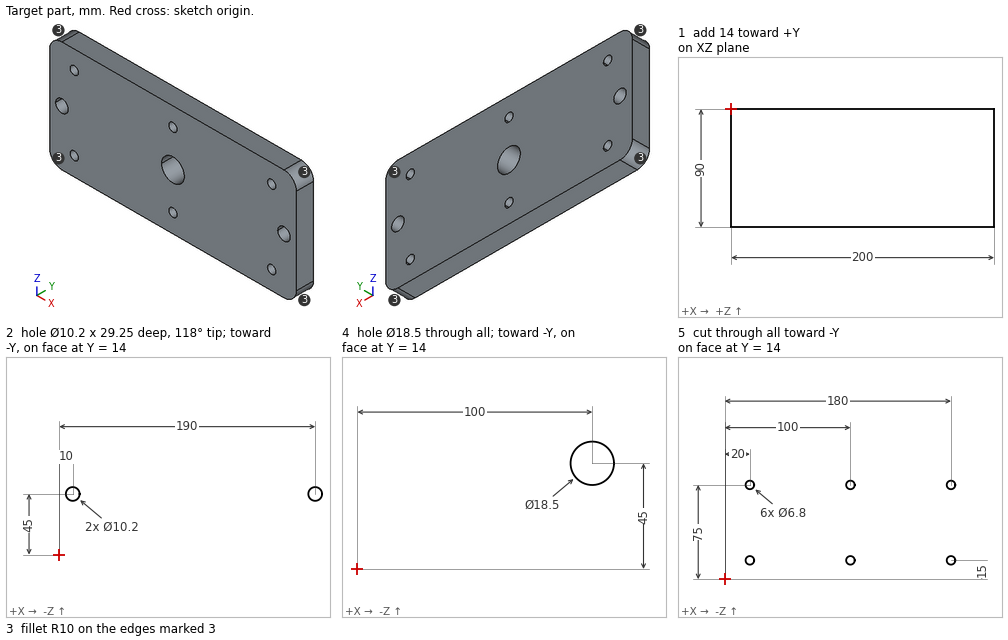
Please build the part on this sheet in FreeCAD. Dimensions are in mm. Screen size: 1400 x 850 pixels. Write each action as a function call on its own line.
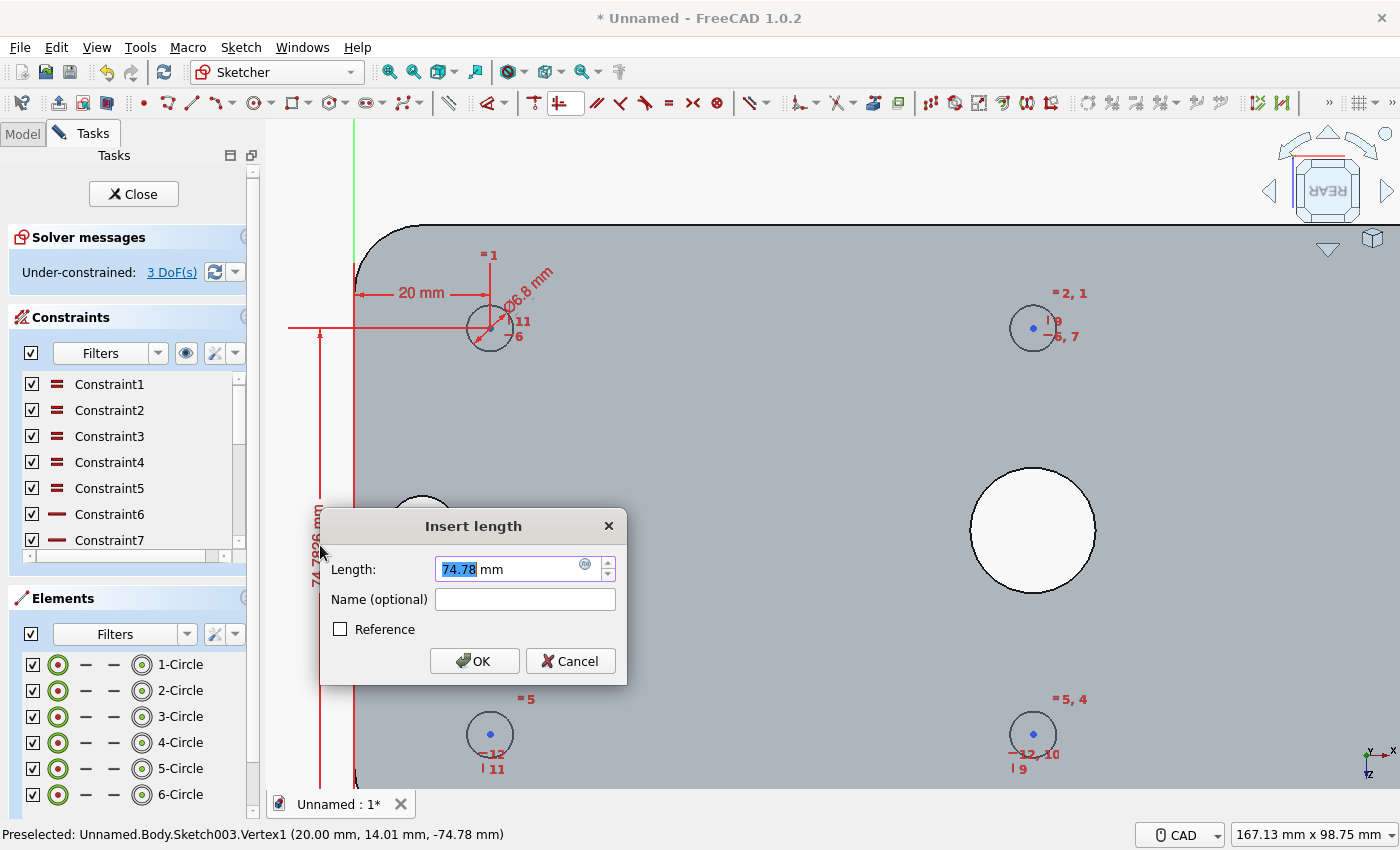
text(75)
key(Return)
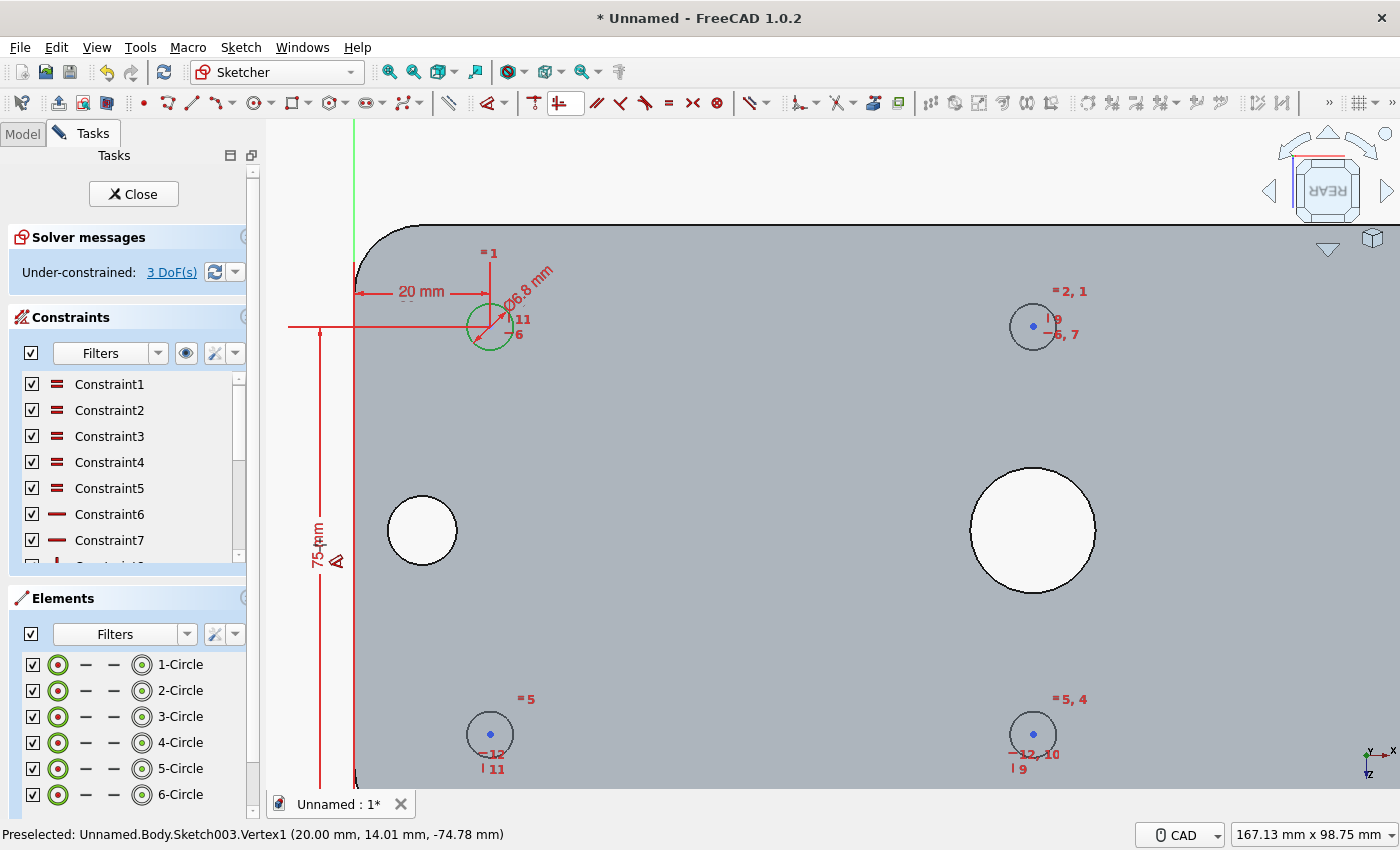
scroll(506, 313, down, 3)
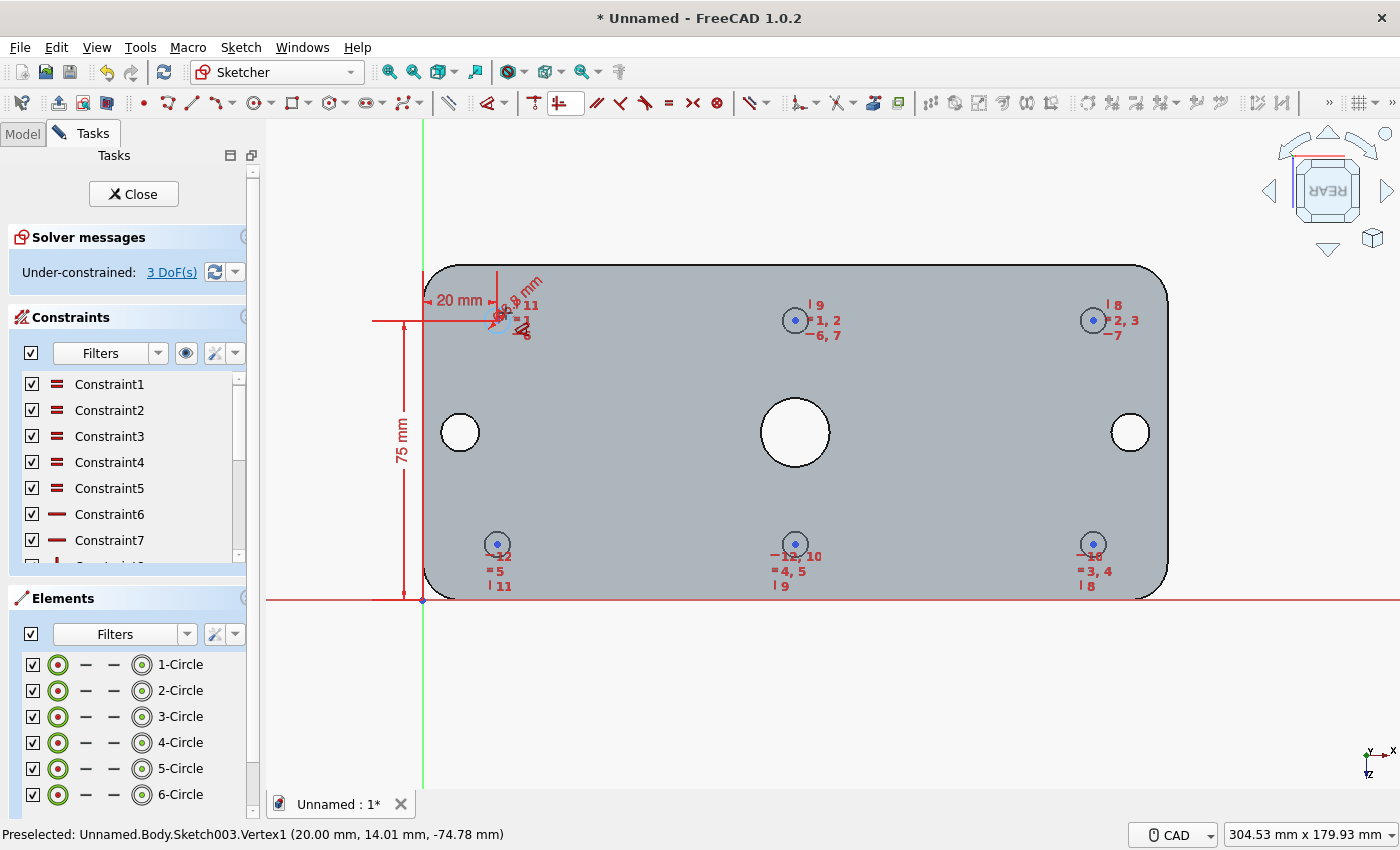
click(1093, 545)
click(389, 572)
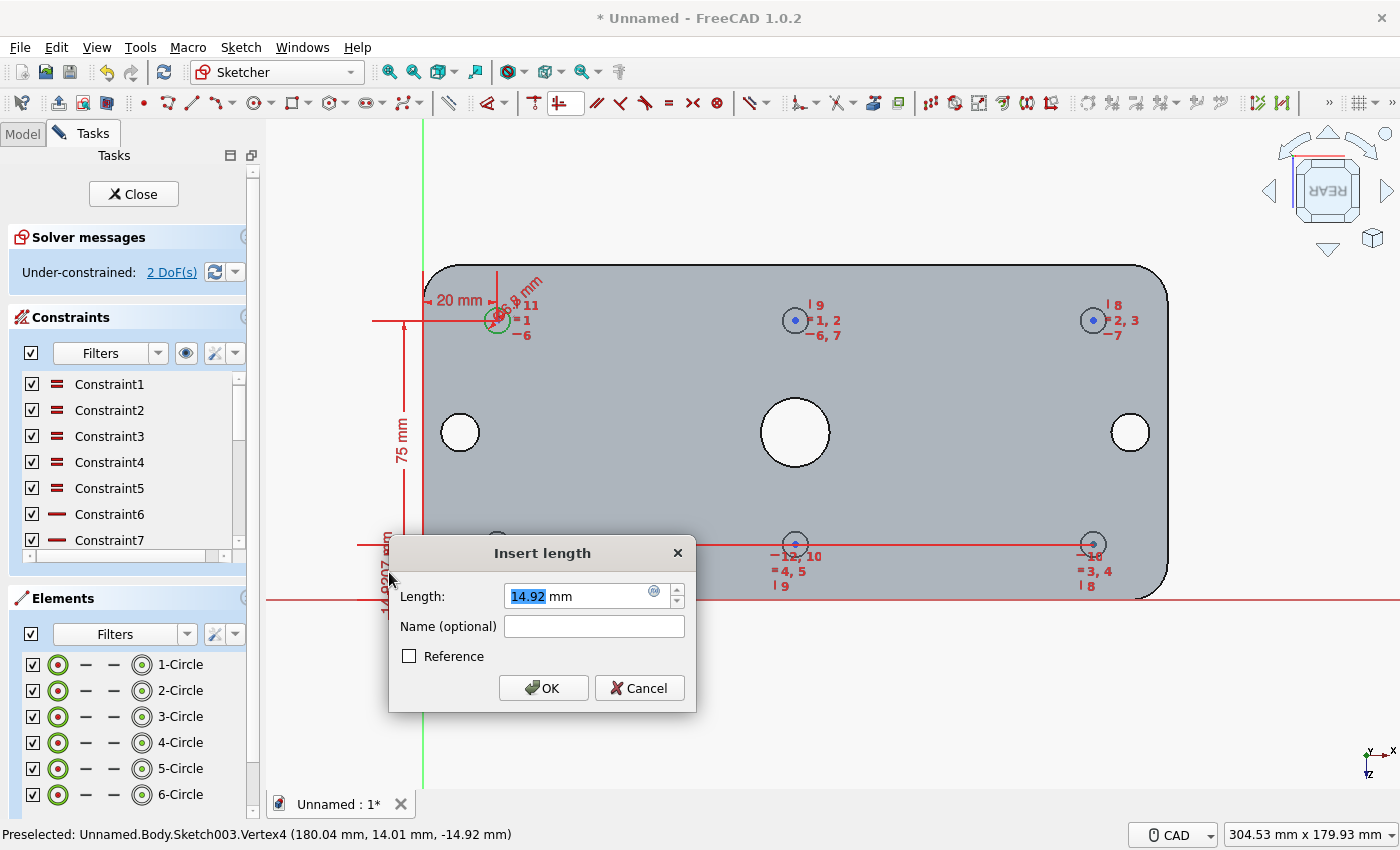
text(15)
key(Return)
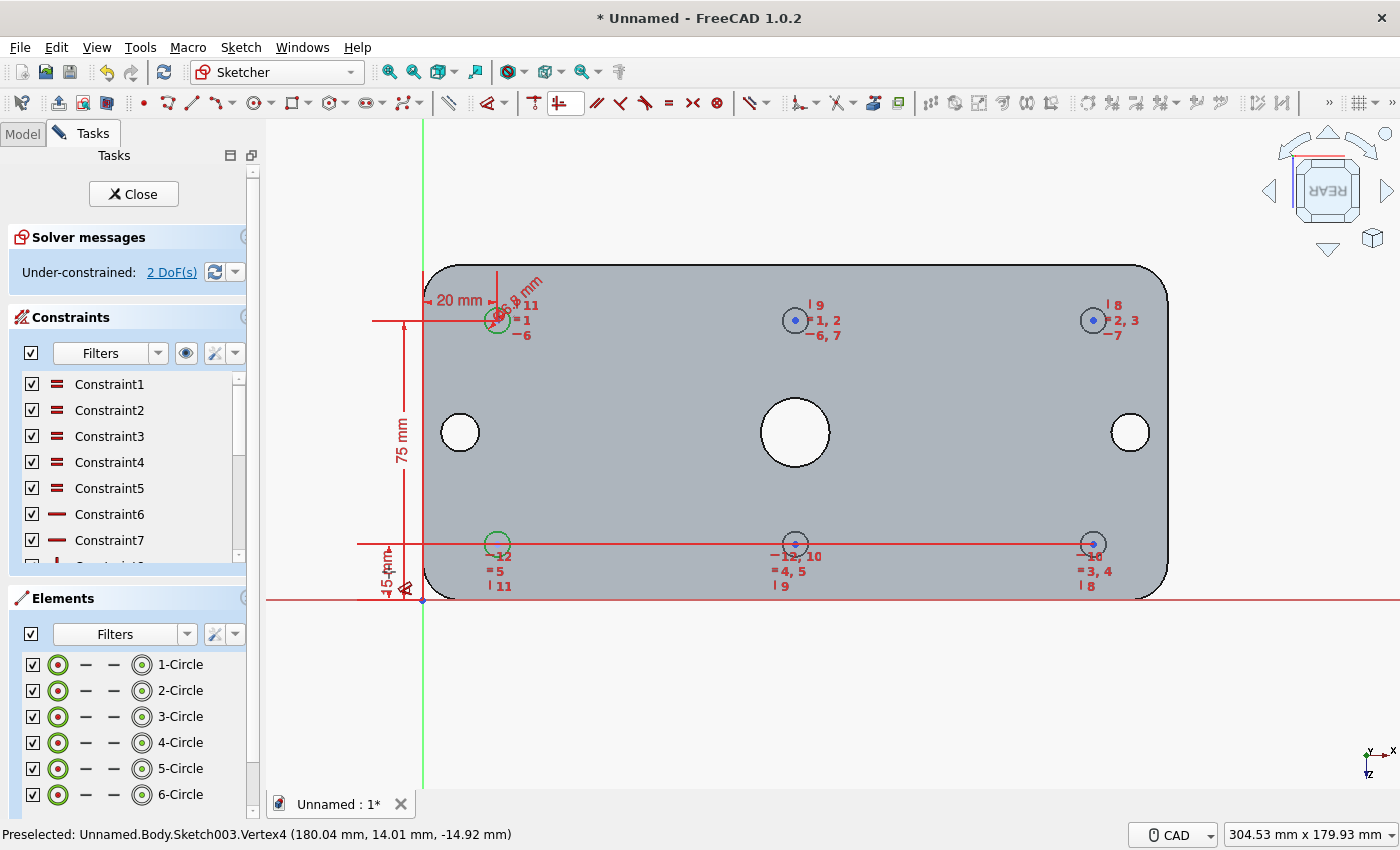
click(795, 321)
click(609, 634)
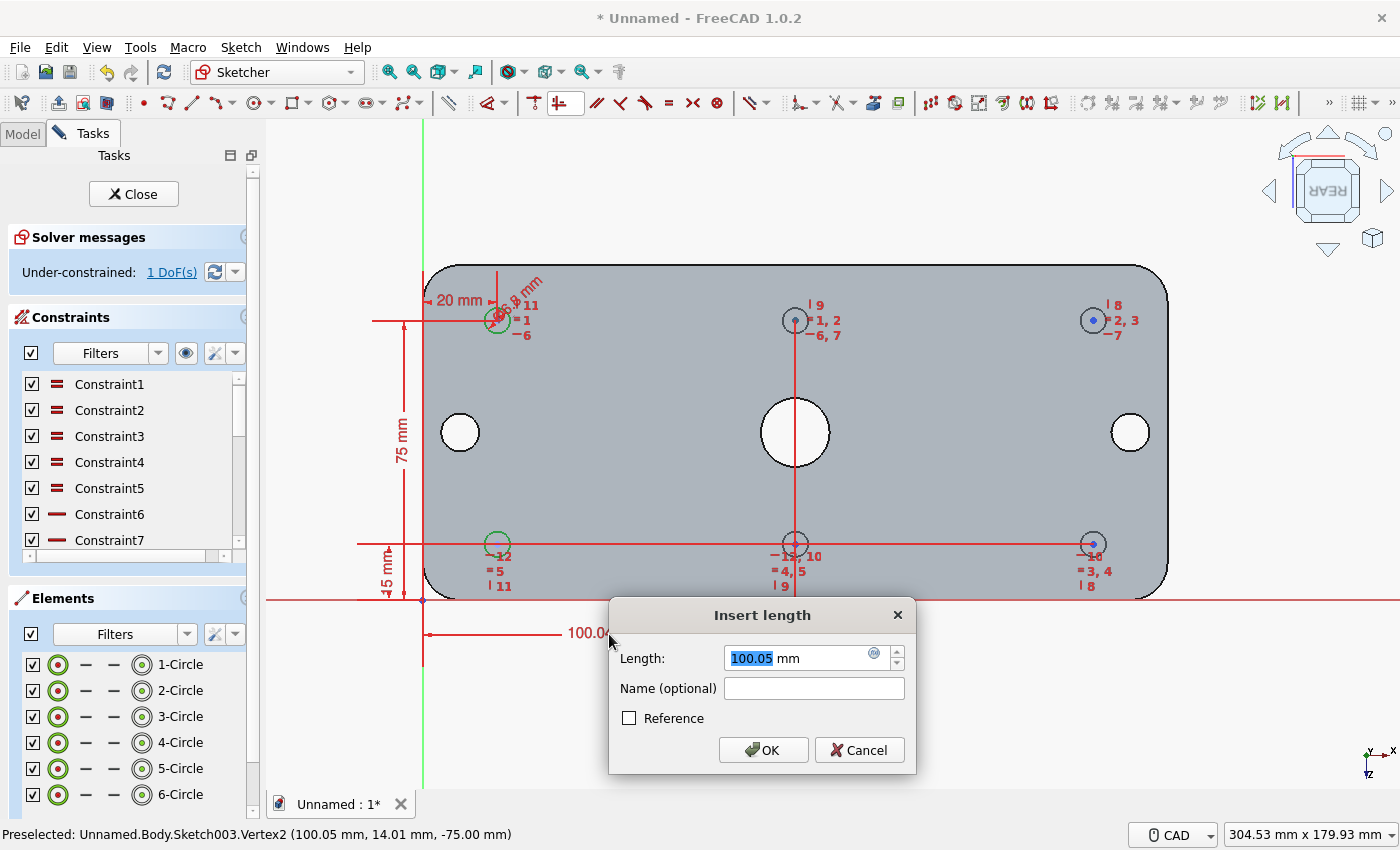
text(100)
key(Return)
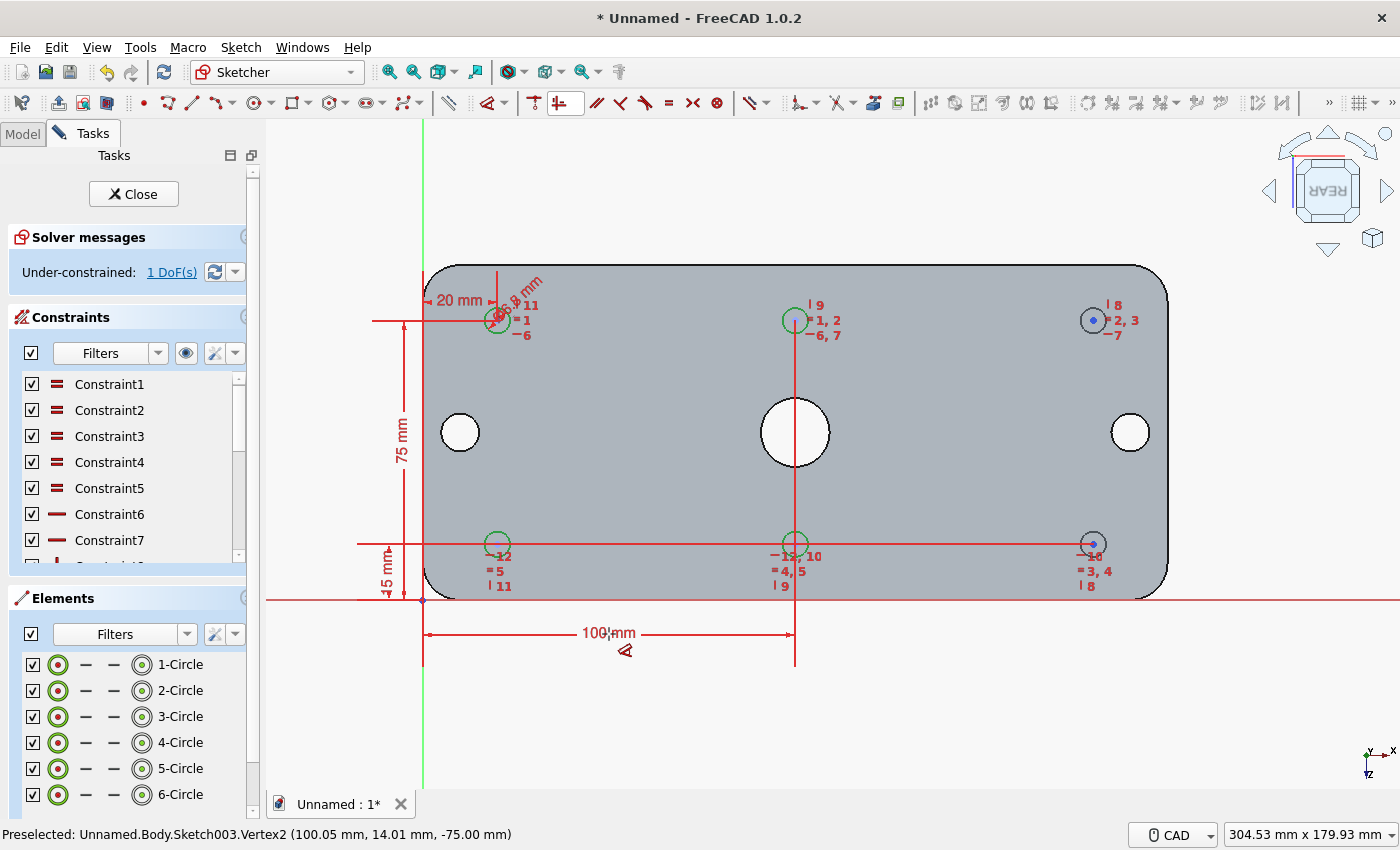
click(1093, 321)
click(758, 634)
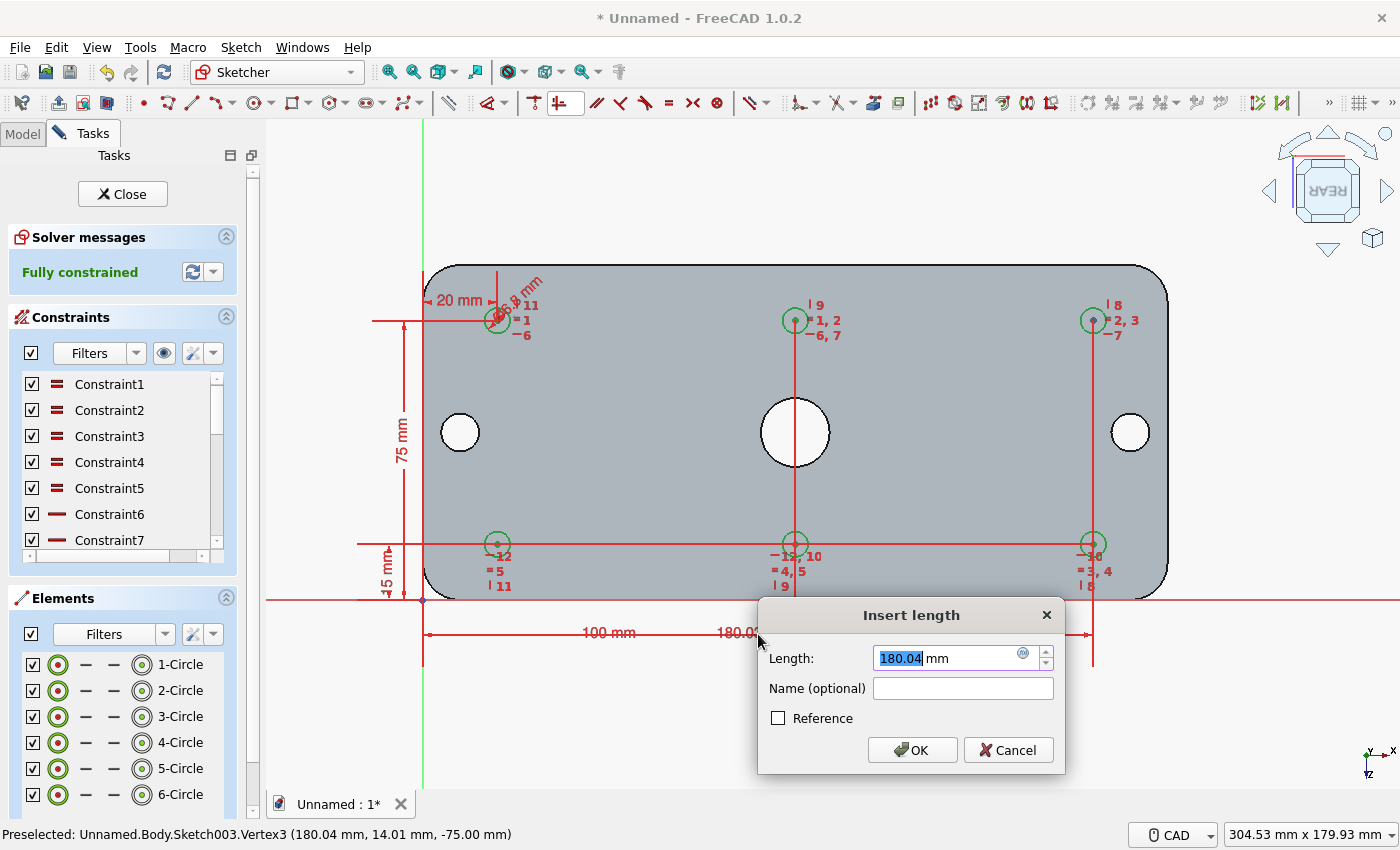
text(180)
key(Return)
key(Escape)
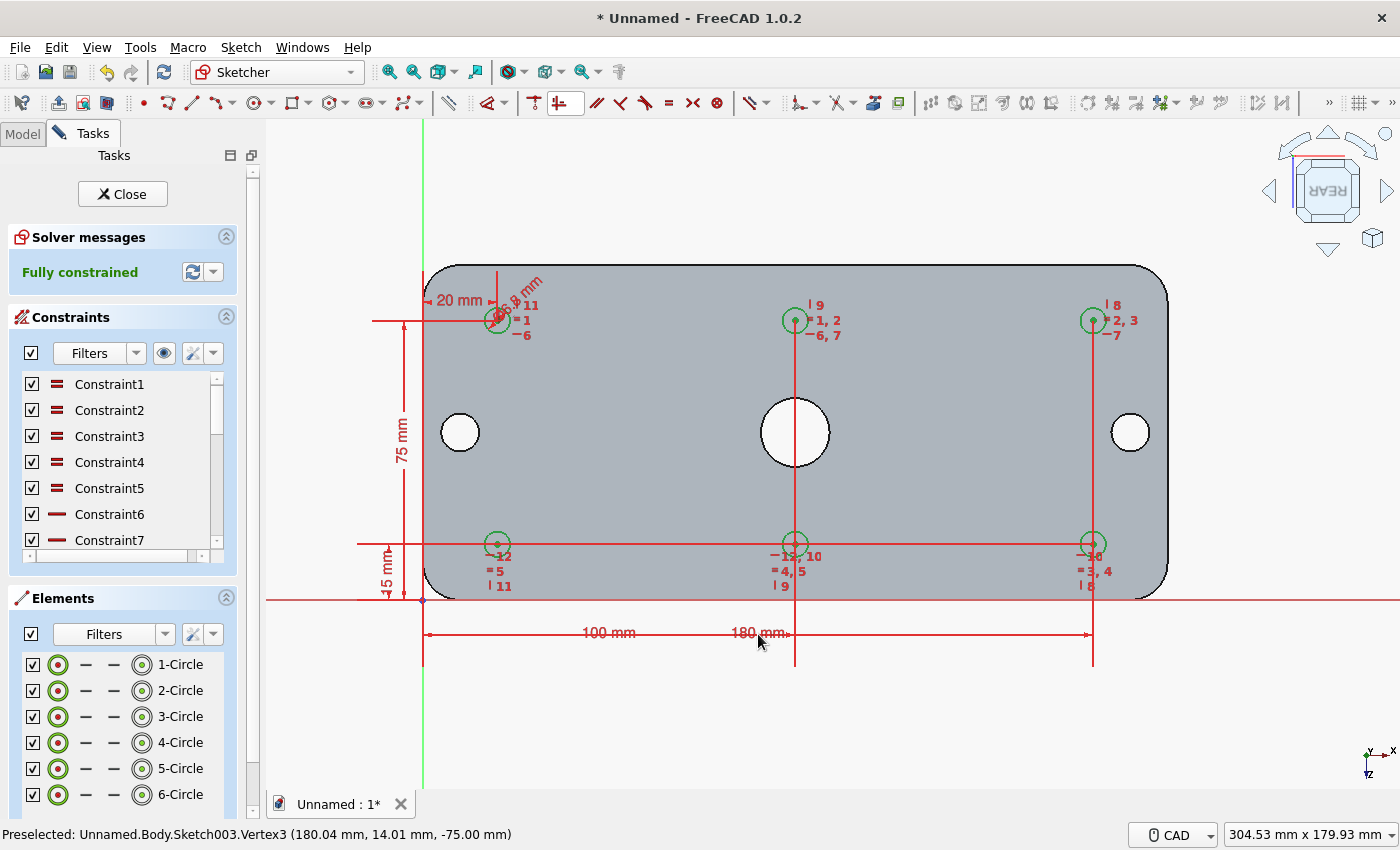
click(123, 194)